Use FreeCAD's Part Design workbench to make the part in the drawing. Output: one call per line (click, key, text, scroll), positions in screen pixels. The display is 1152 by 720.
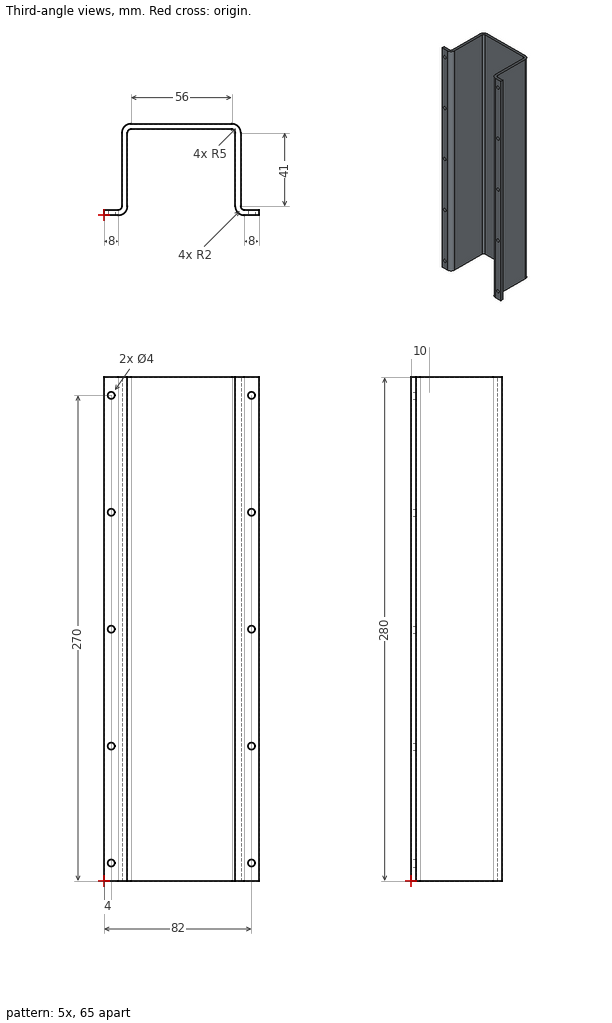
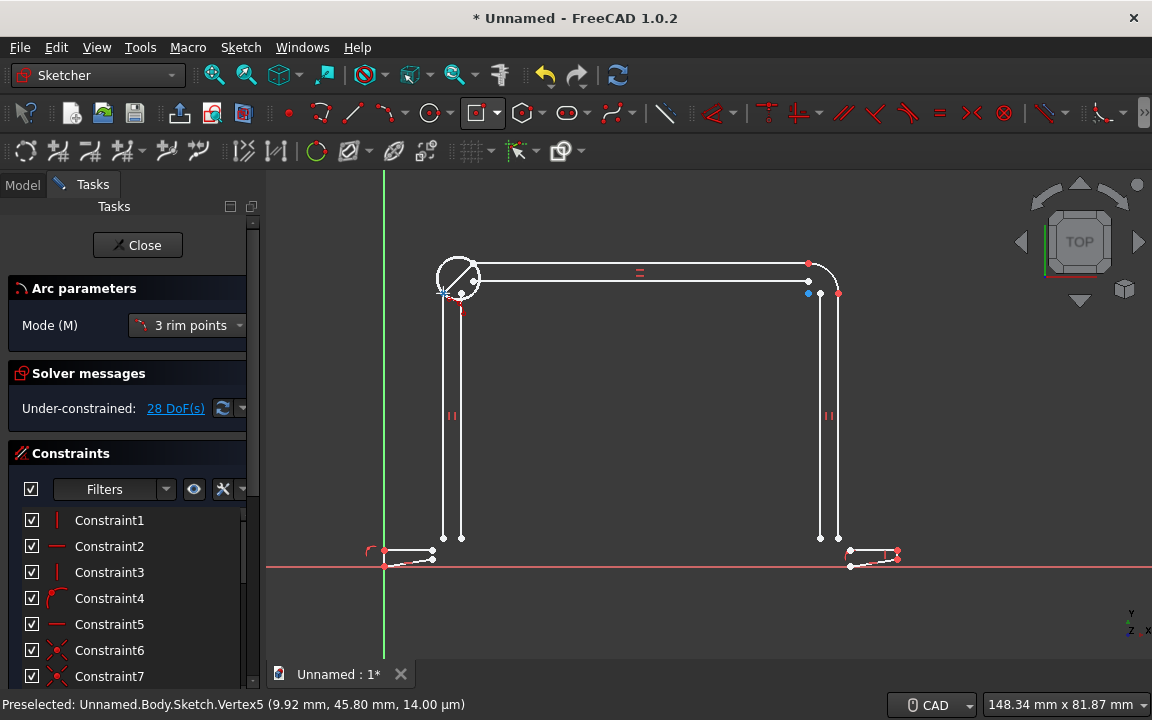
scroll(453, 271, up, 3)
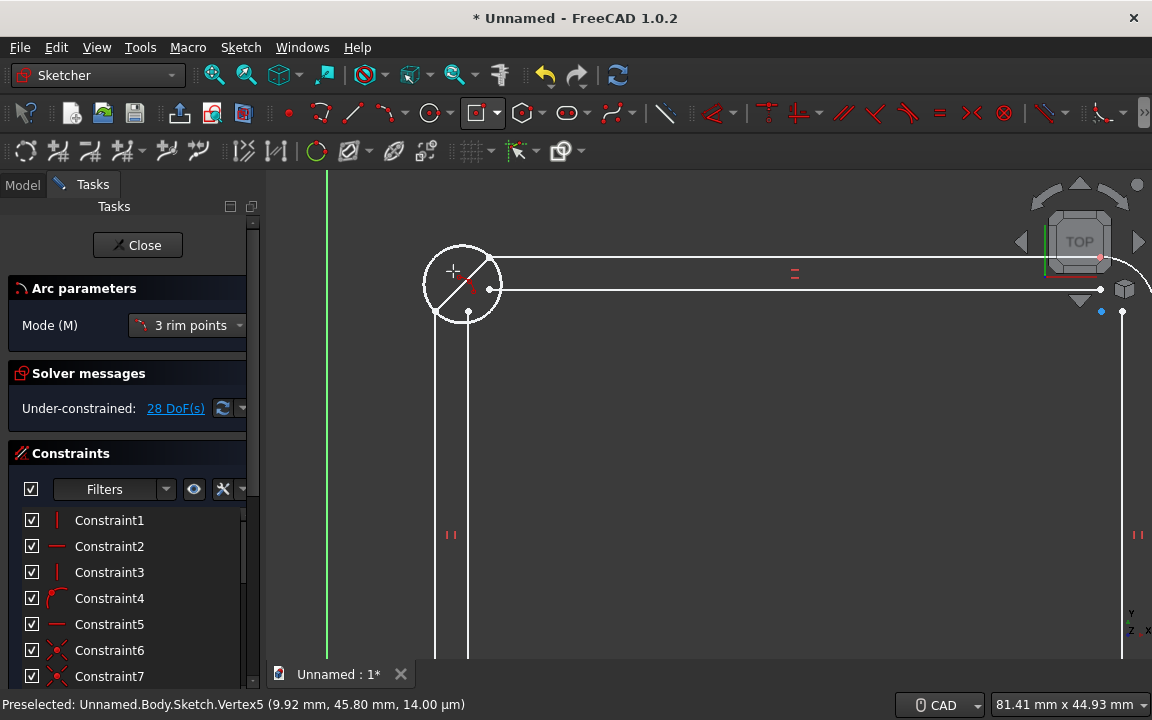
click(452, 271)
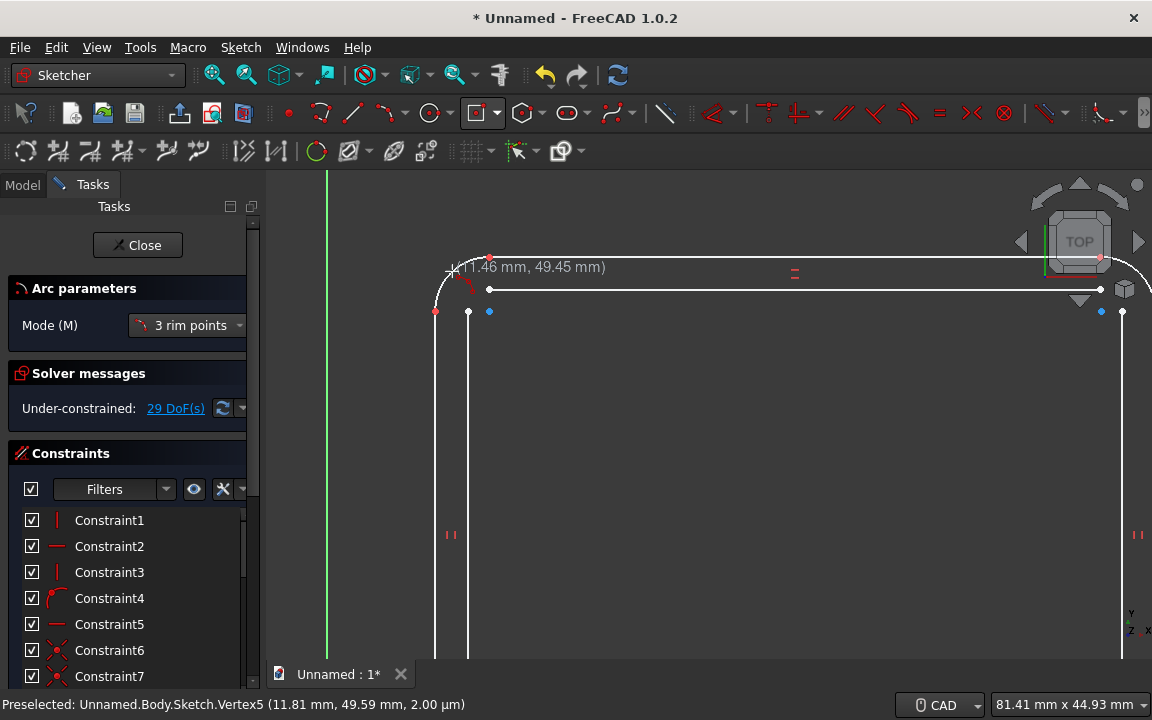
scroll(452, 271, down, 3)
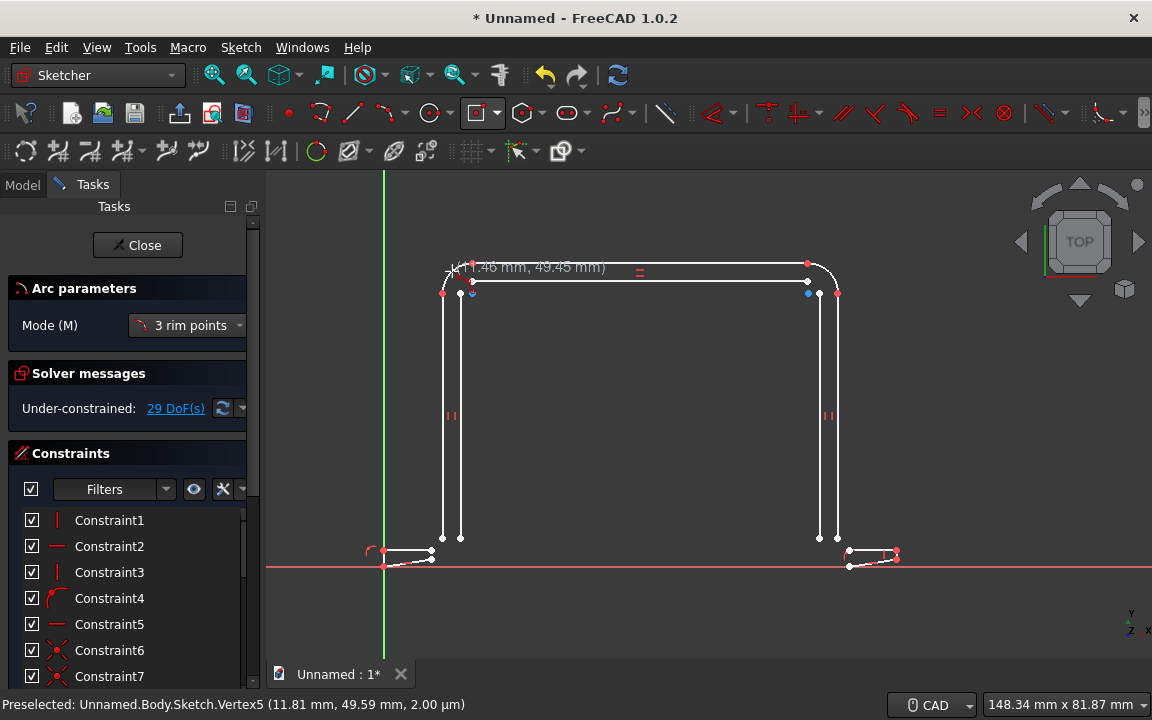
click(443, 538)
click(432, 550)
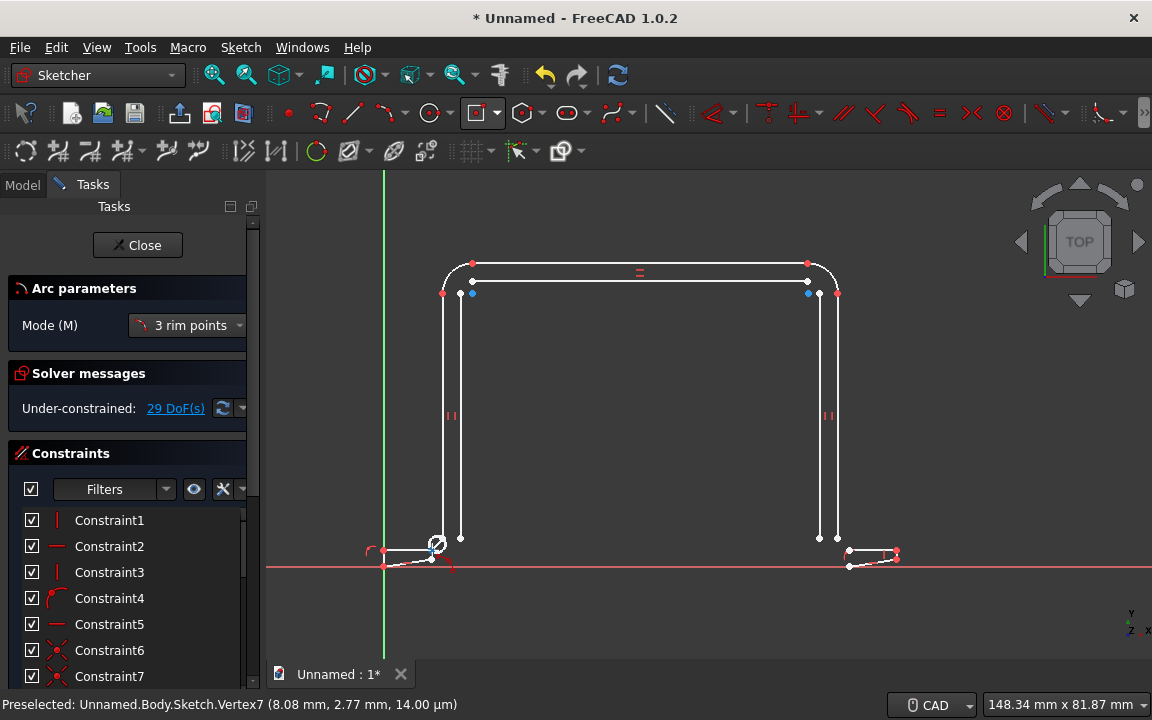
scroll(440, 546, up, 8)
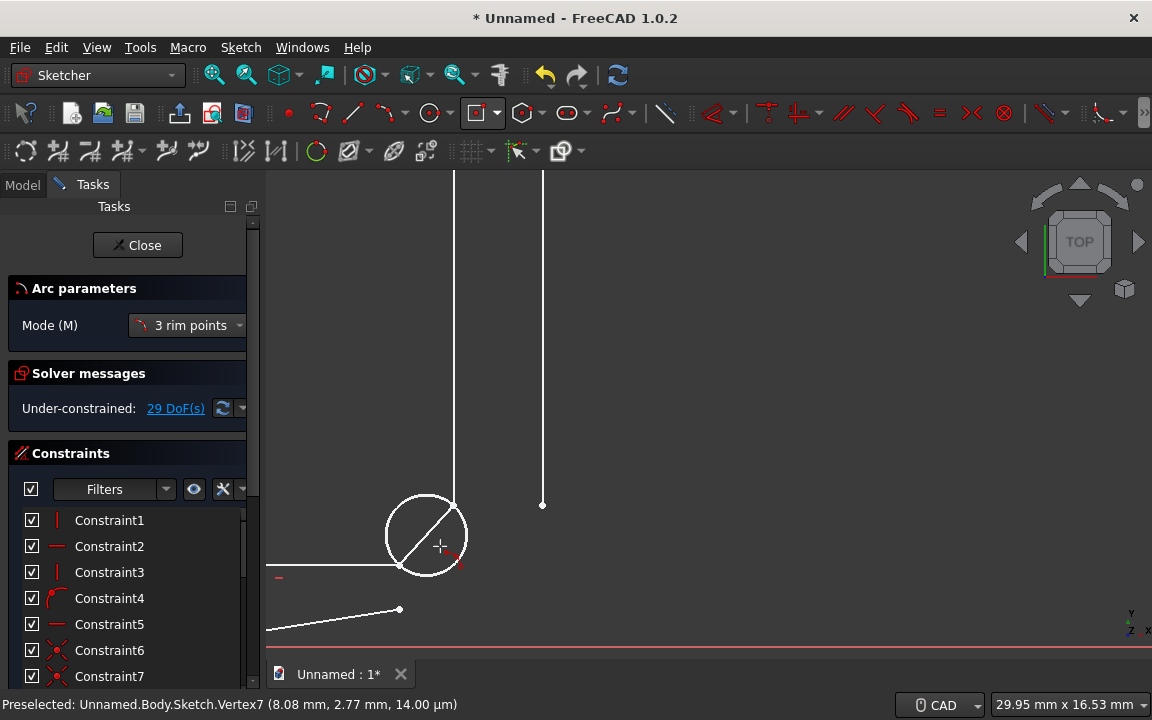
click(439, 541)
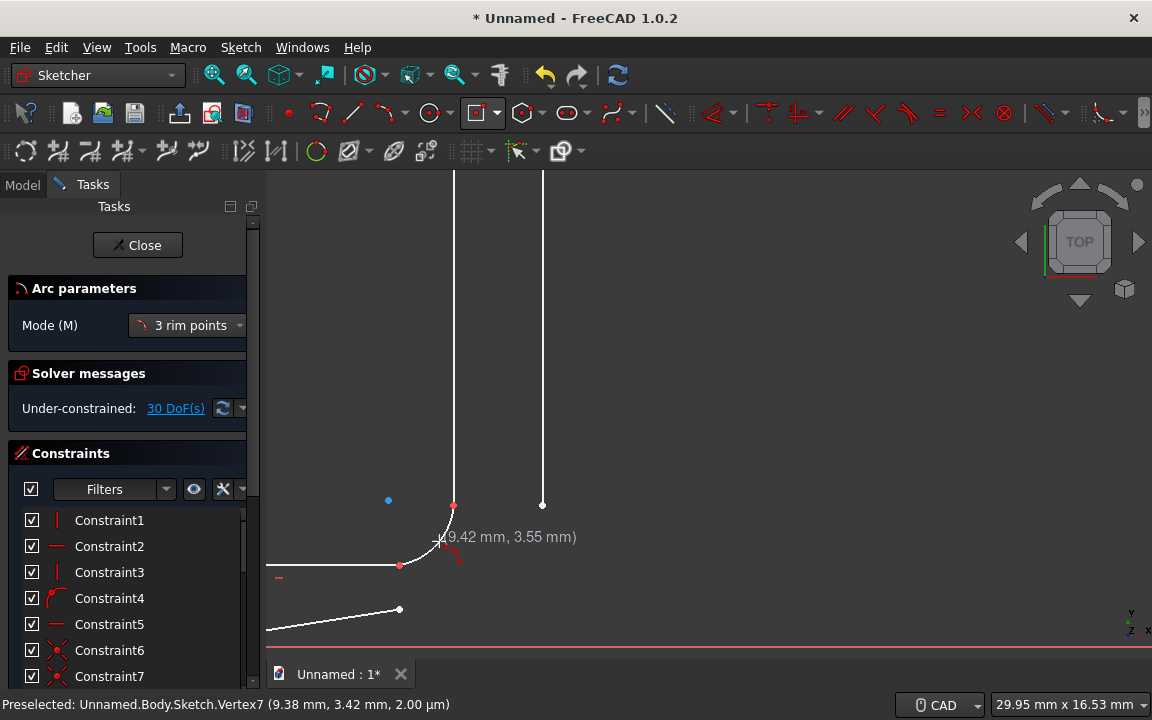
scroll(440, 547, down, 8)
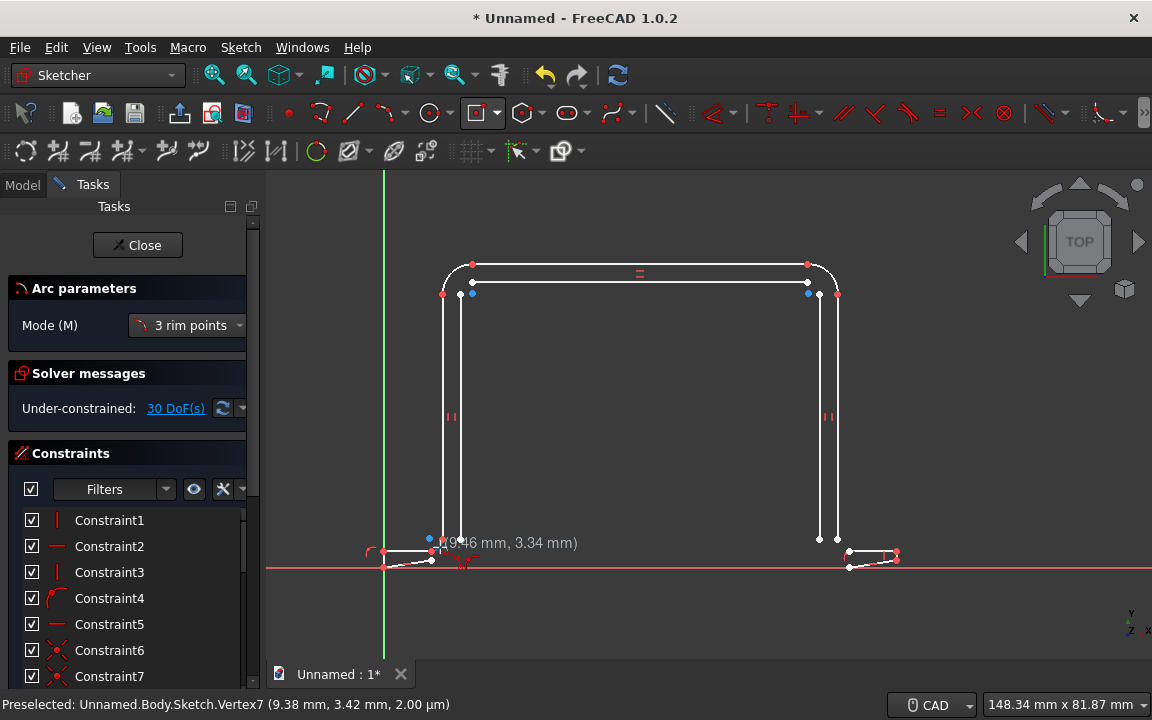
click(432, 560)
click(461, 539)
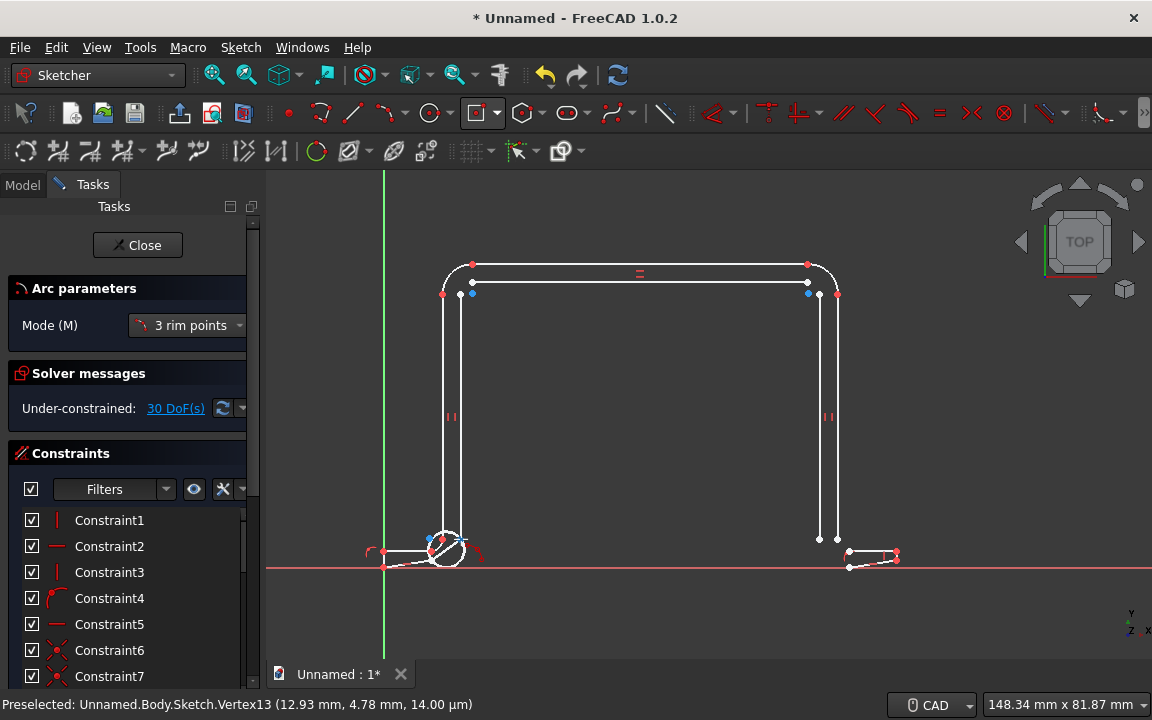
scroll(453, 559, up, 3)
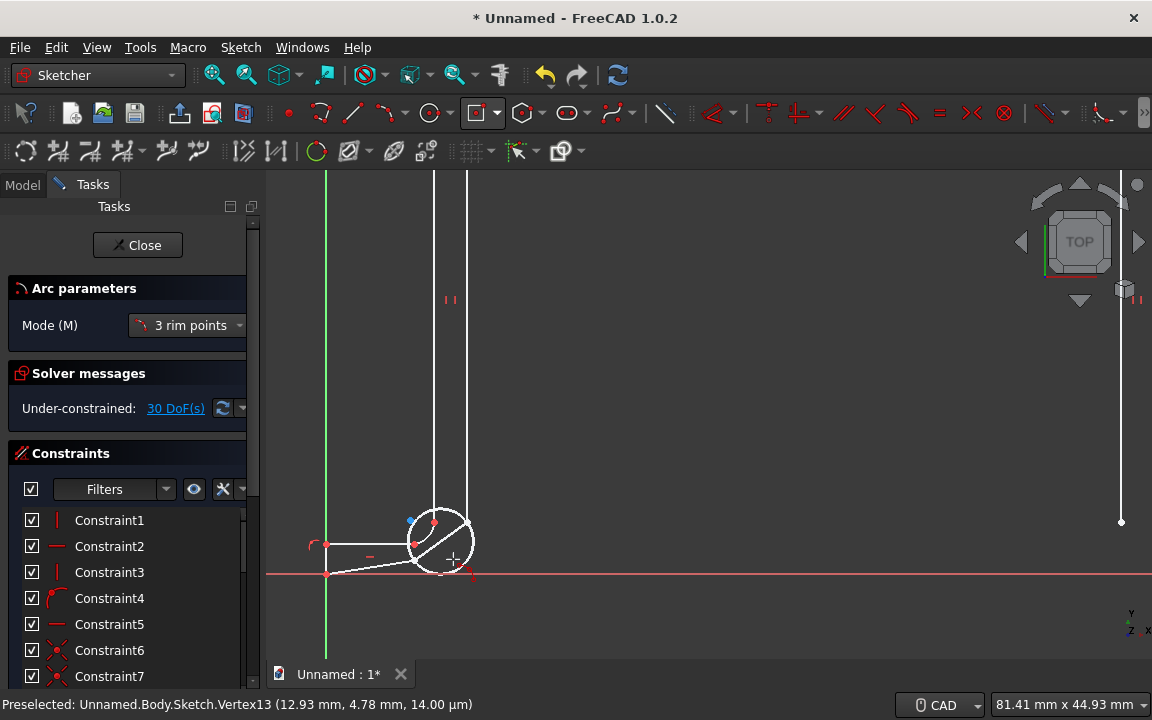
click(452, 558)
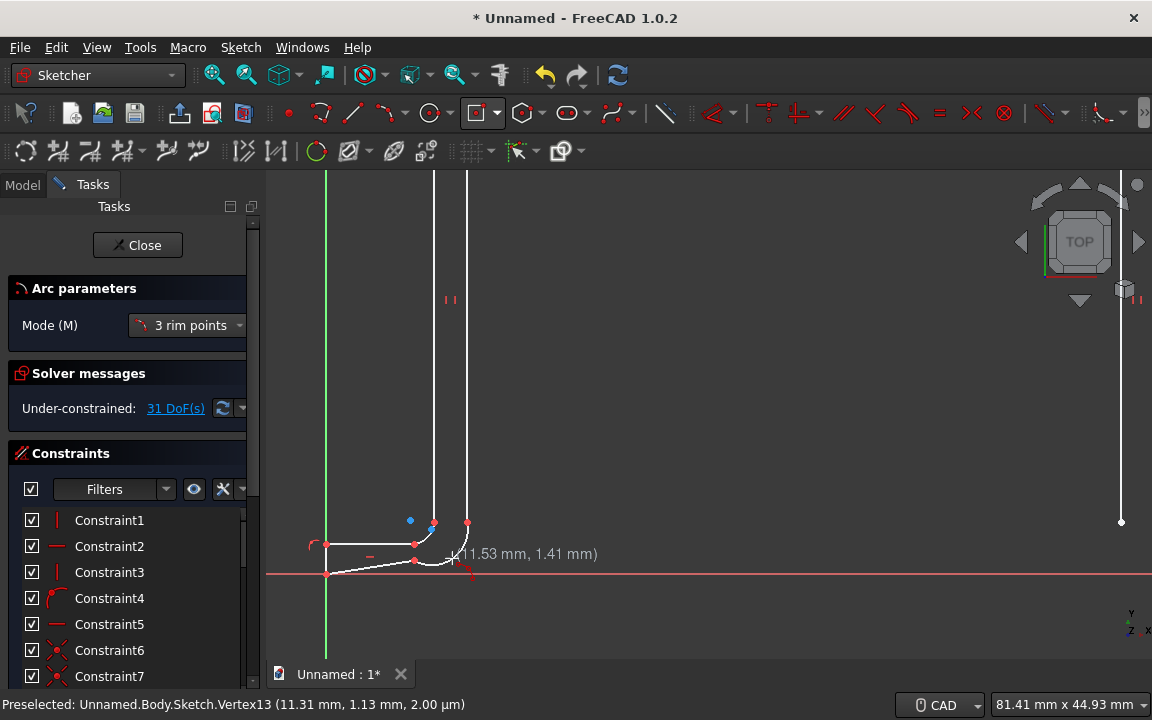
scroll(453, 558, down, 3)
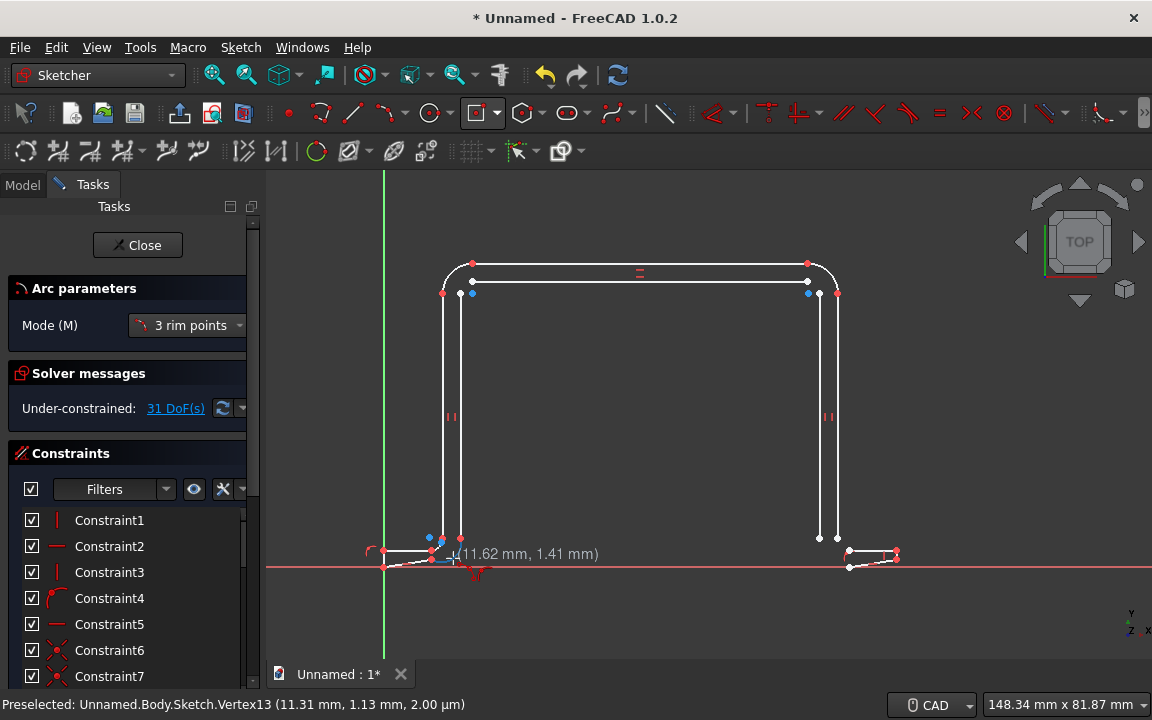
scroll(461, 293, up, 2)